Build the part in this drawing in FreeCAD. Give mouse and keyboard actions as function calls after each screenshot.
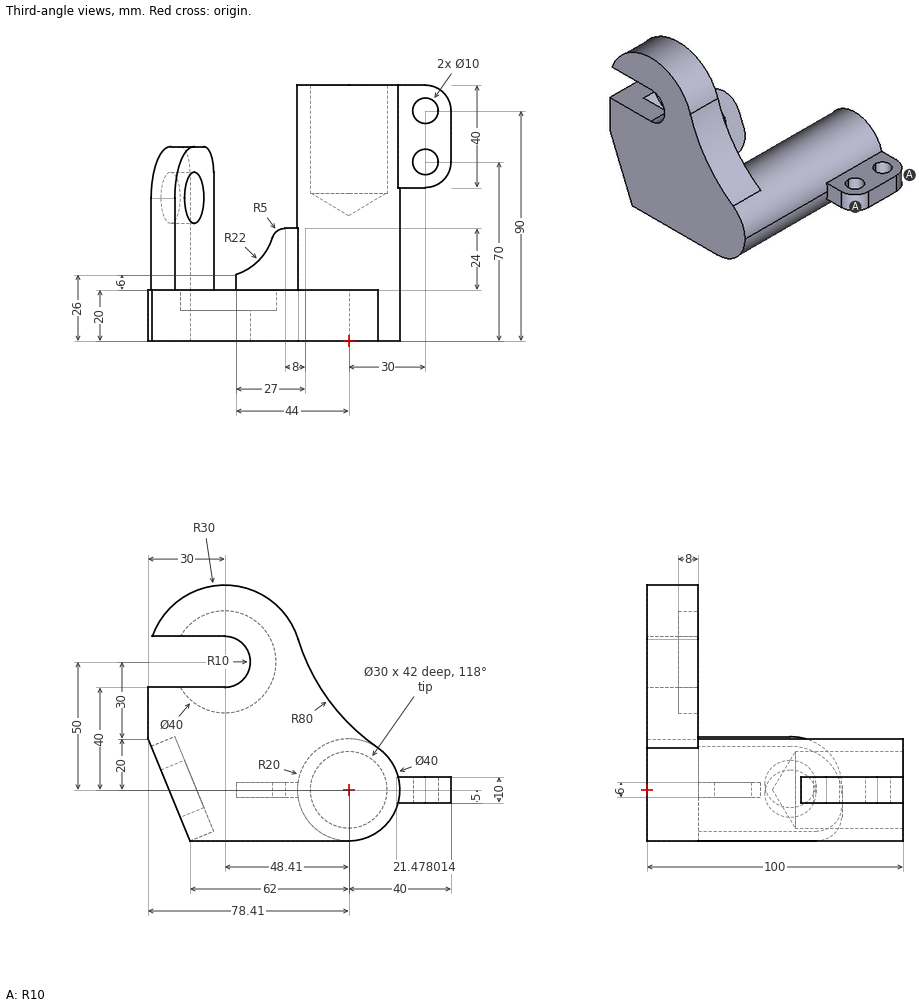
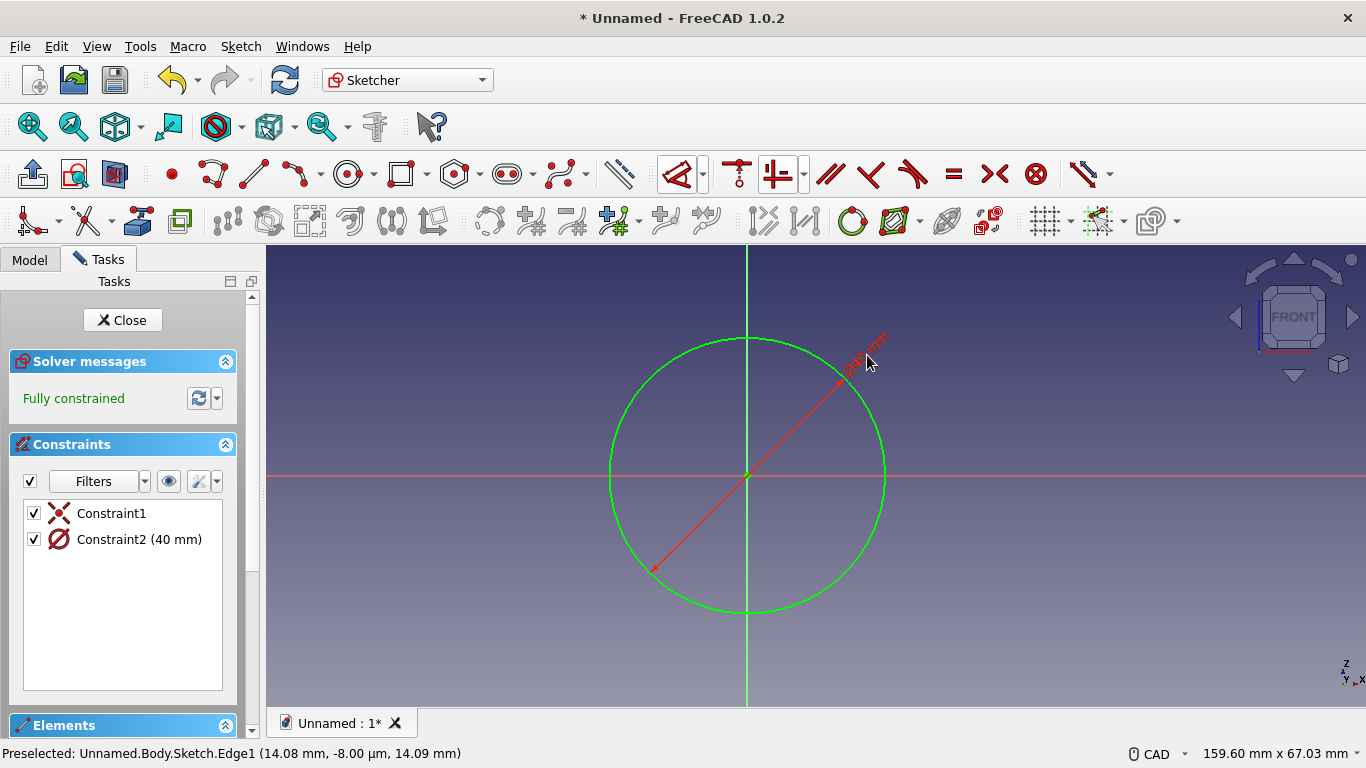
click(123, 320)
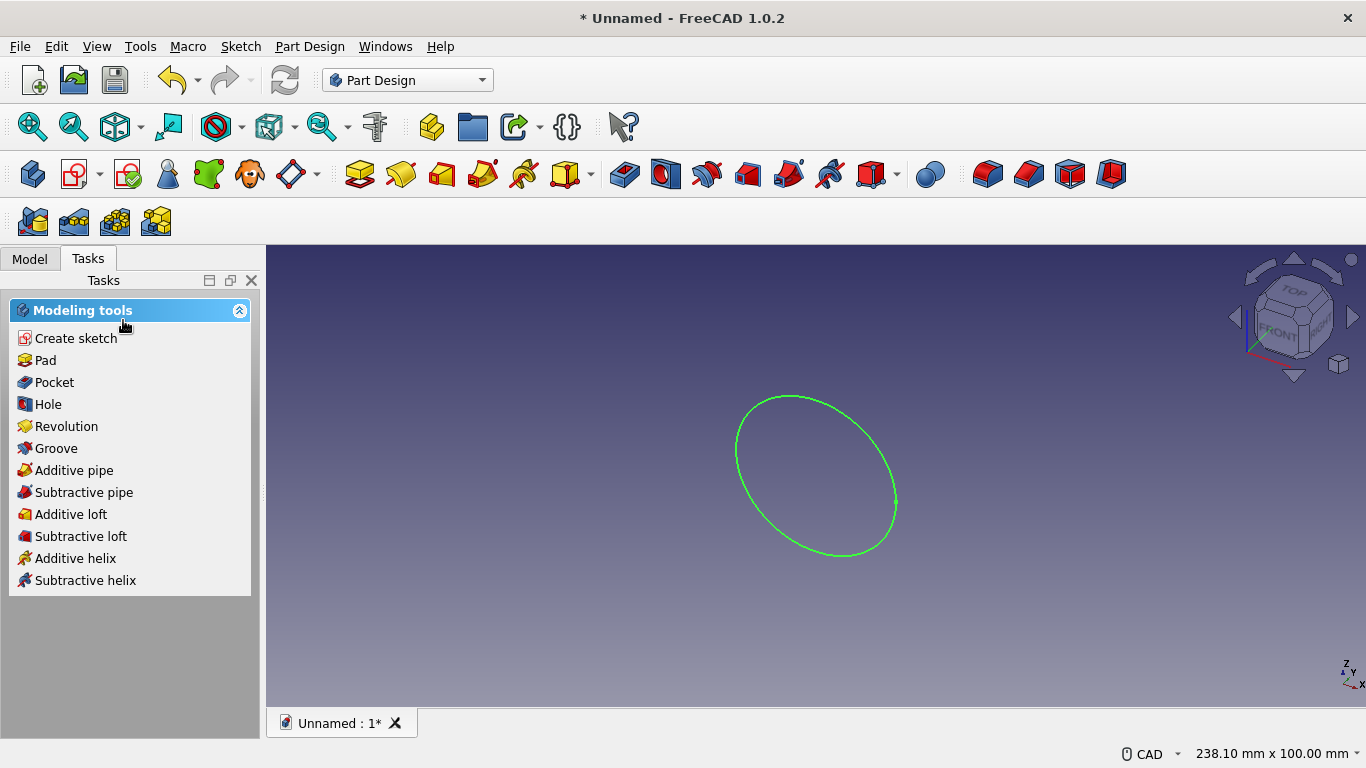
click(360, 174)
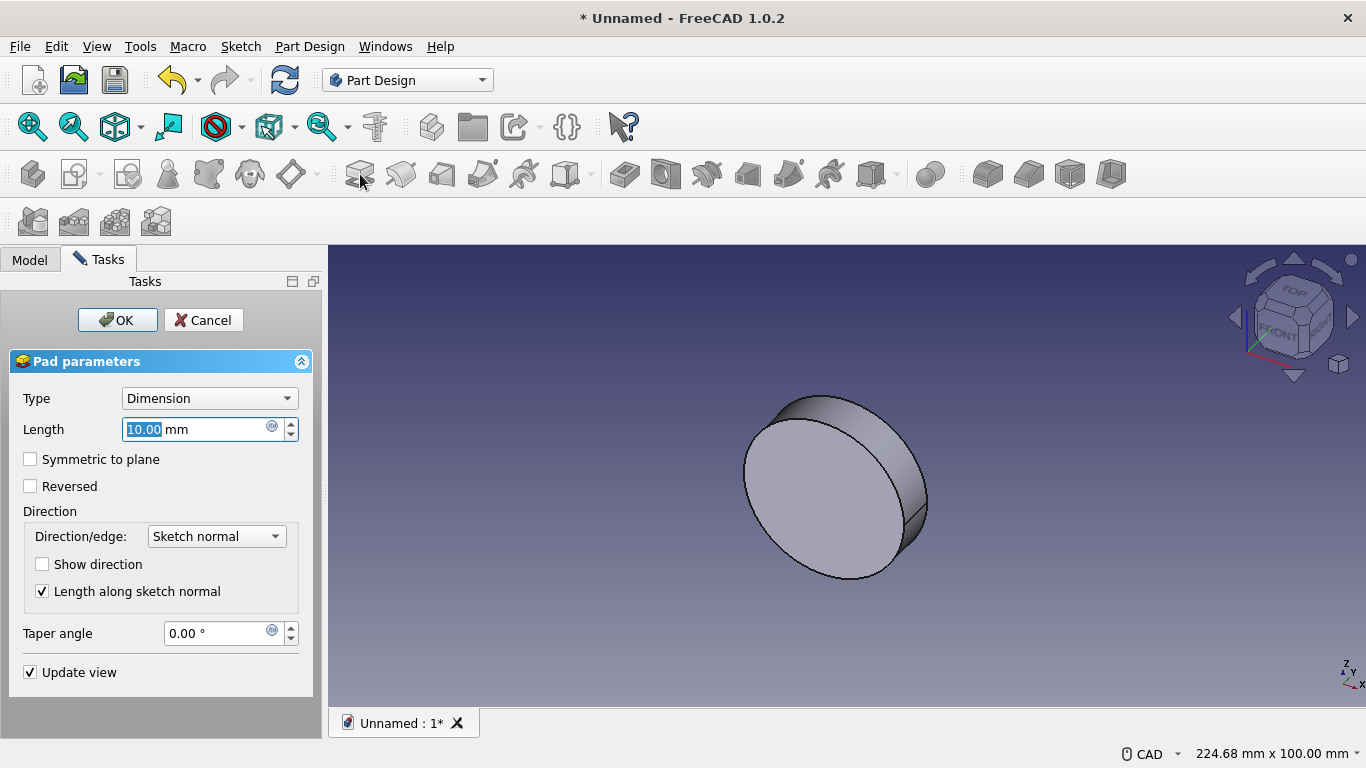
text(100)
key(Tab)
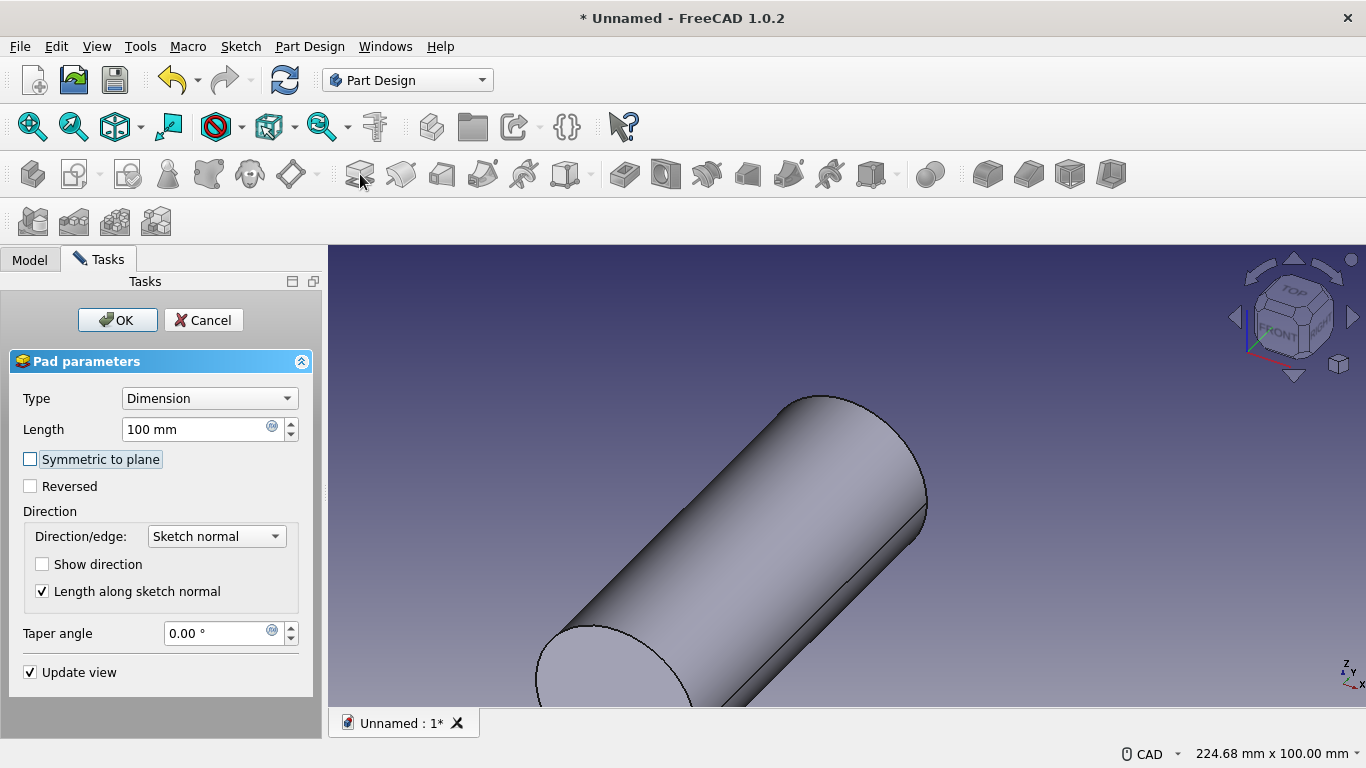
click(31, 486)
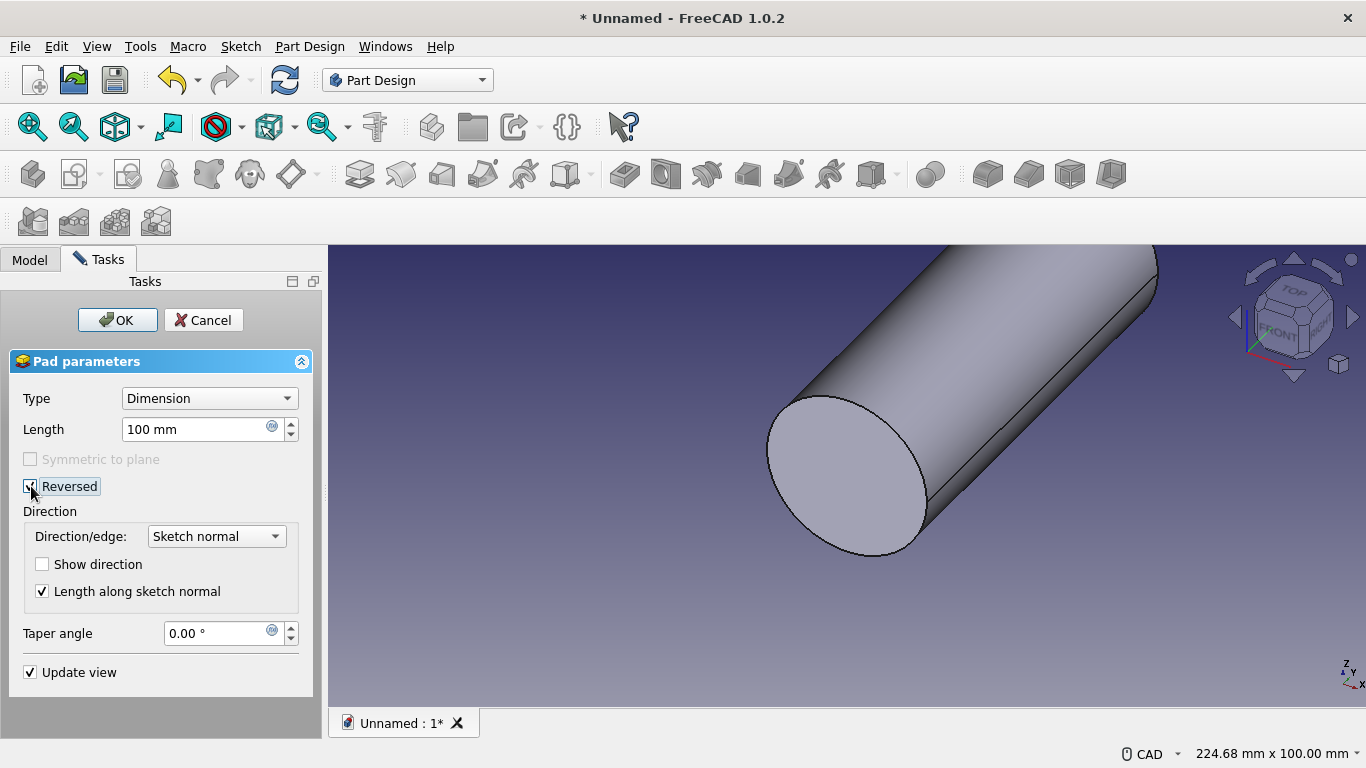
click(118, 320)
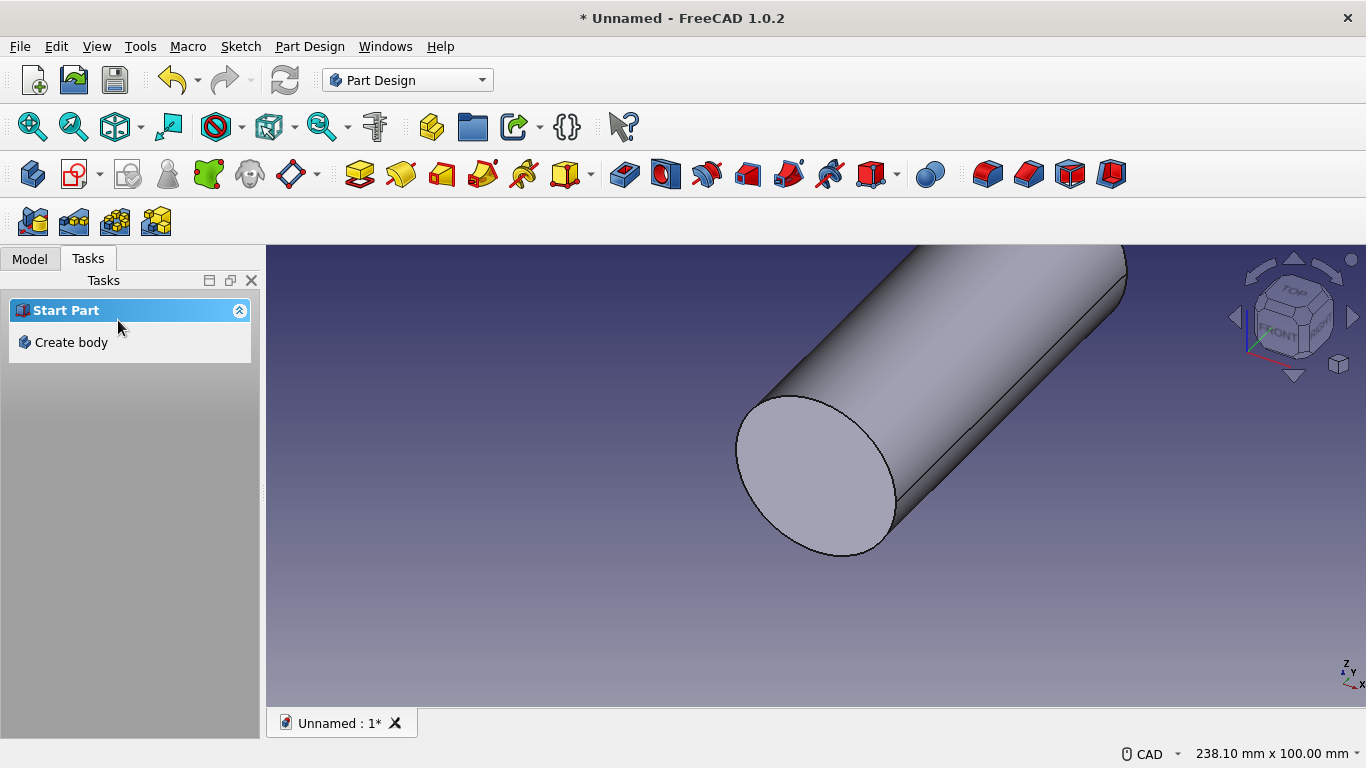
click(33, 128)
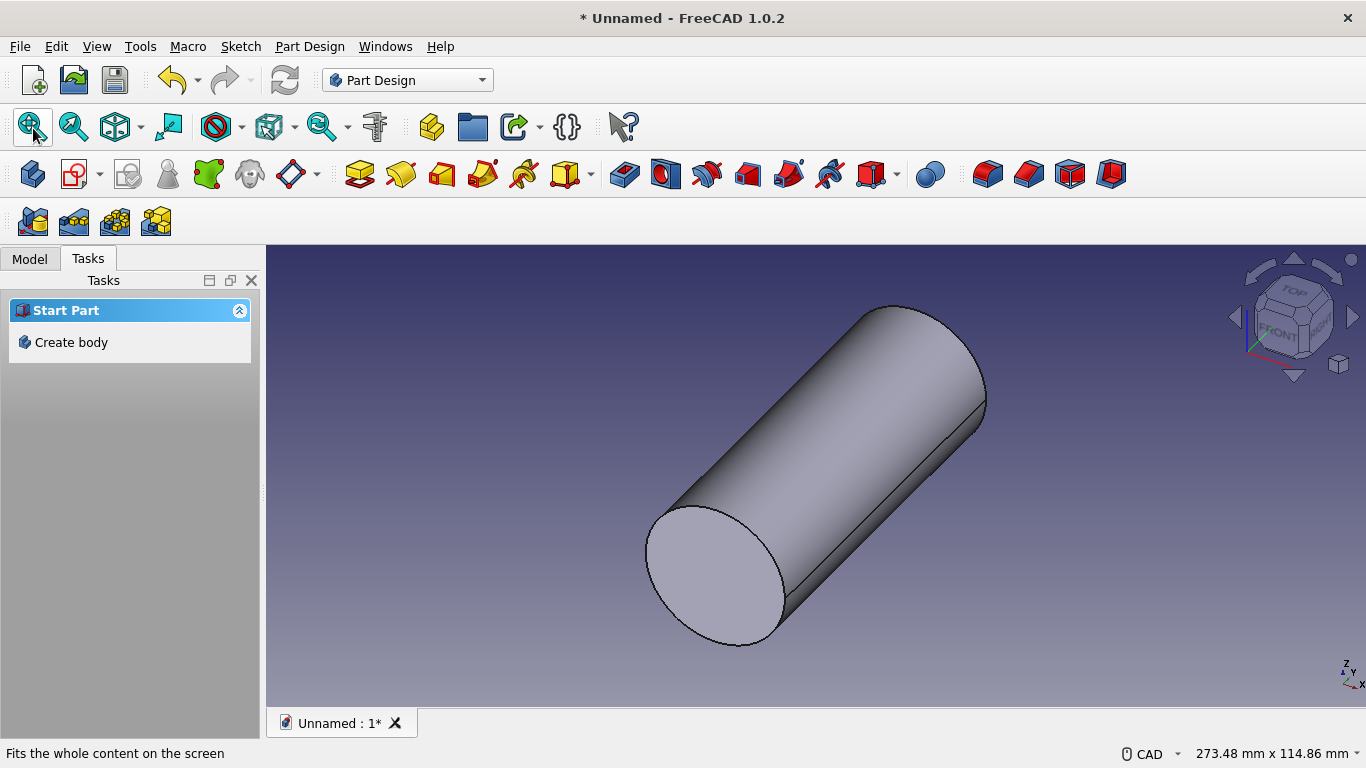
click(74, 174)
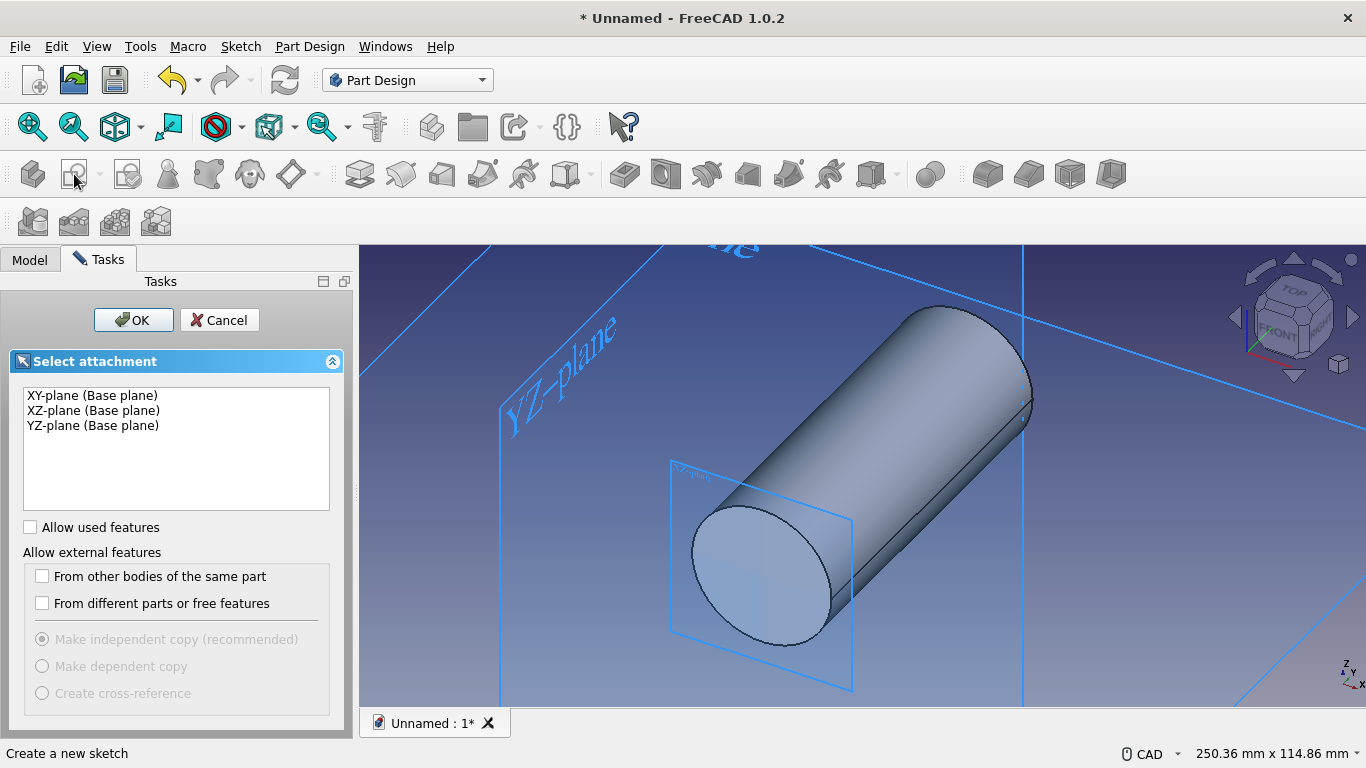
click(84, 410)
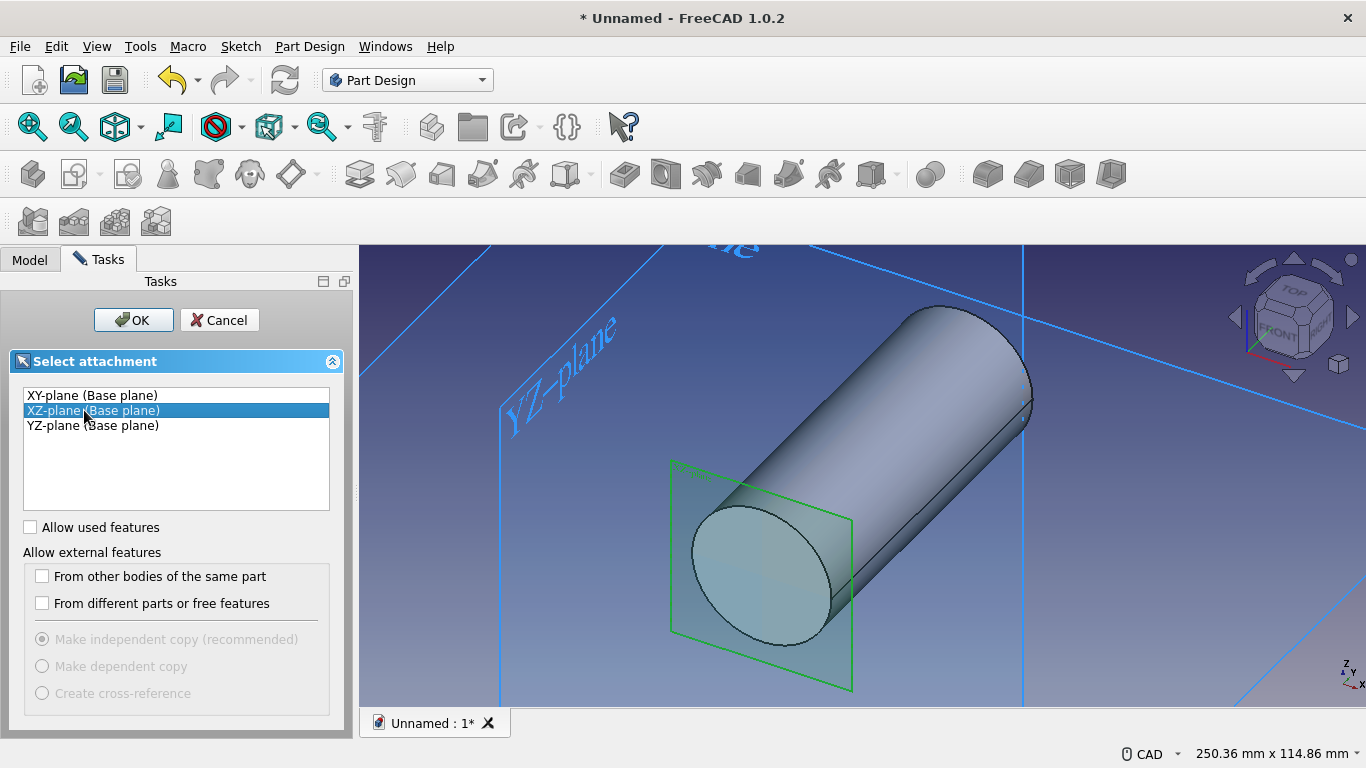
click(134, 320)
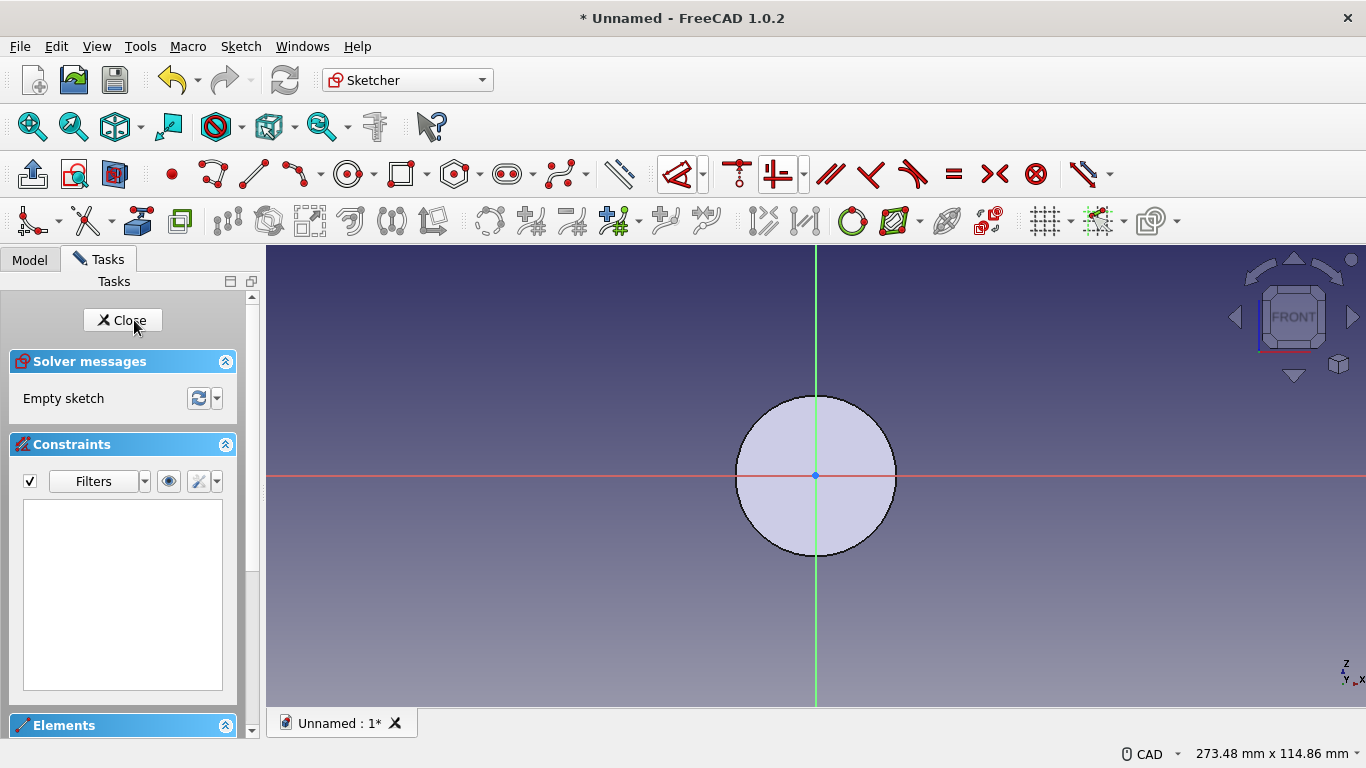
scroll(883, 679, down, 2)